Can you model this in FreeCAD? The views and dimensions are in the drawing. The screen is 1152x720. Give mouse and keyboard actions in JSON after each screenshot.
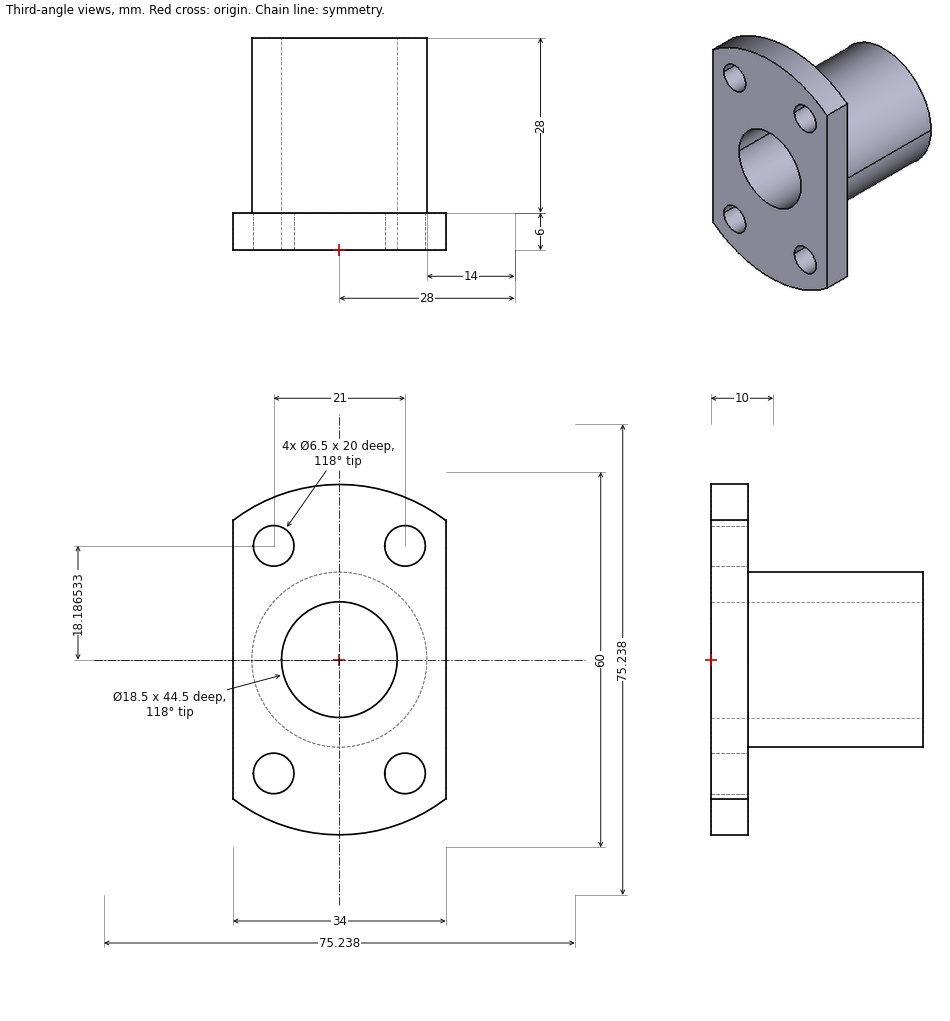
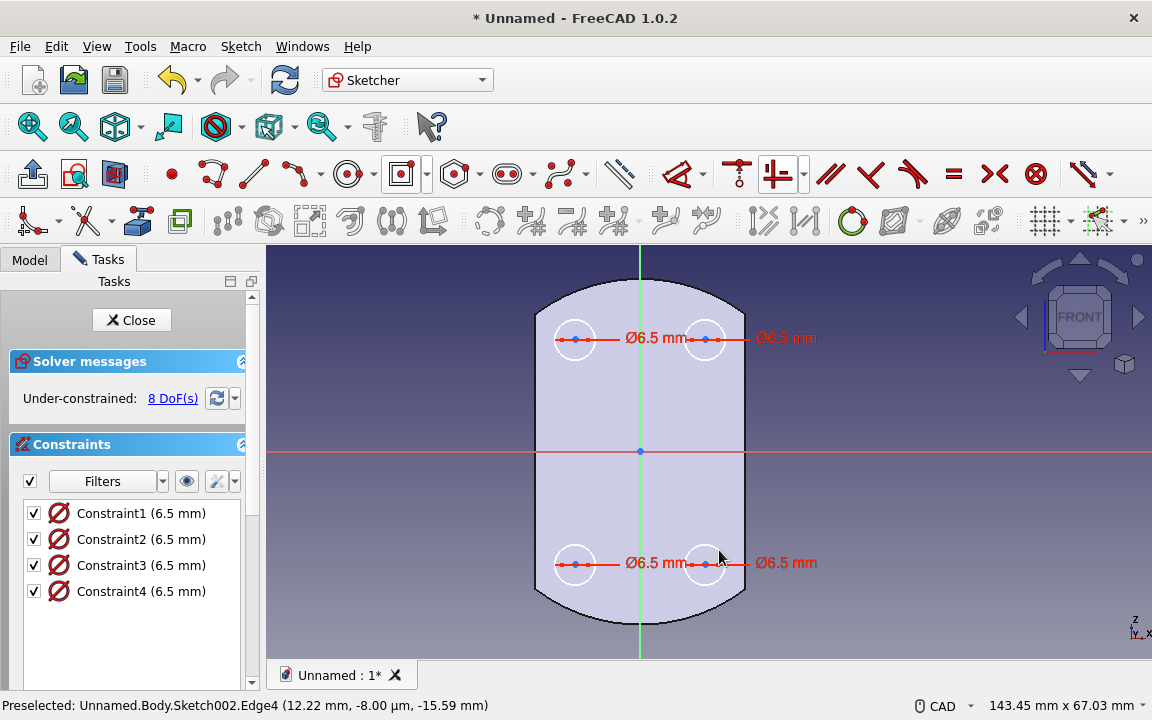
{"action": "left_click", "coordinate": [575, 340]}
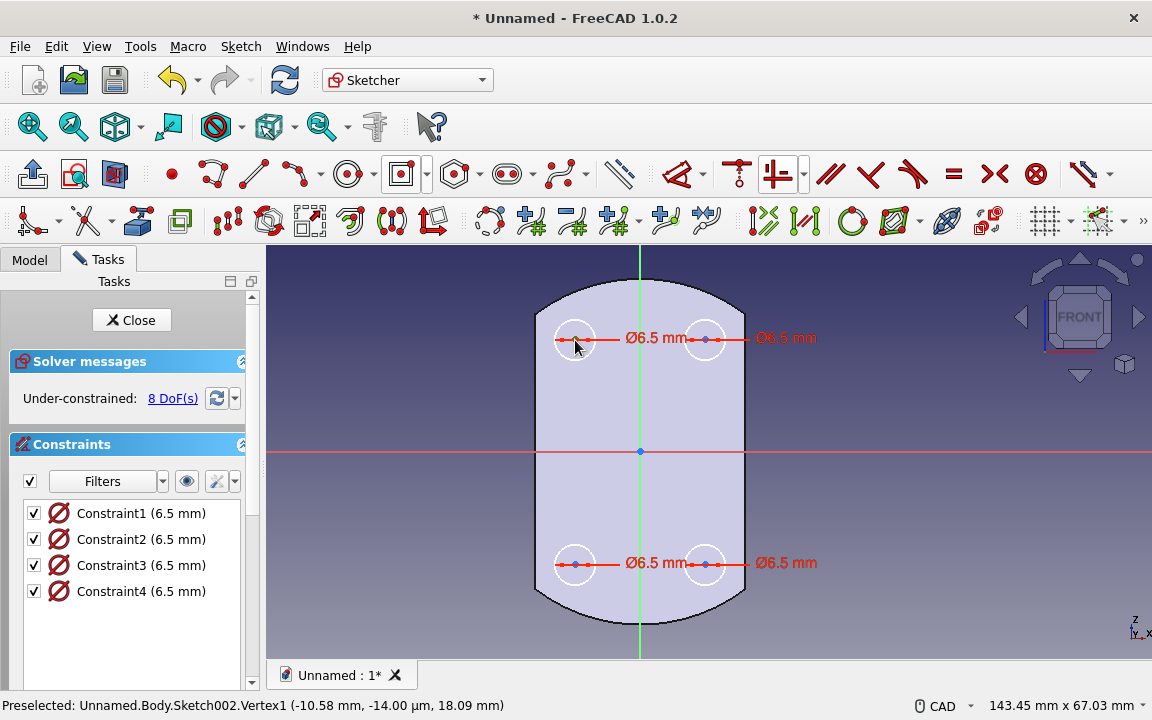
{"action": "left_click", "coordinate": [705, 340]}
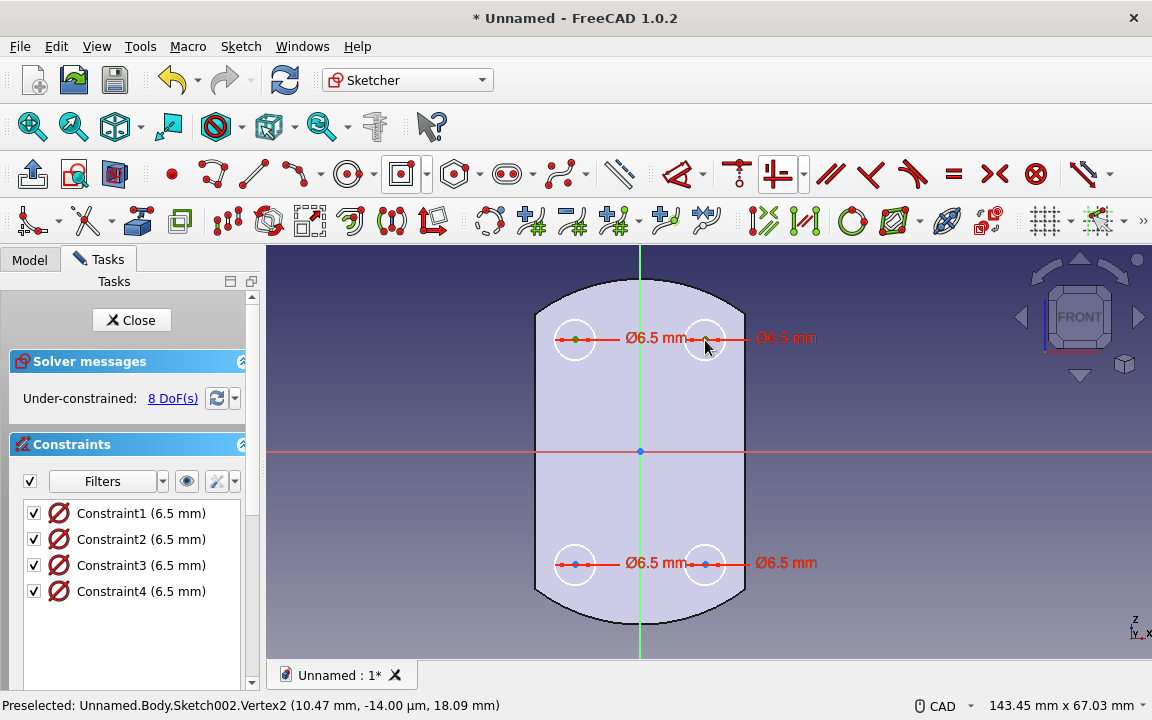
{"action": "left_click", "coordinate": [640, 605]}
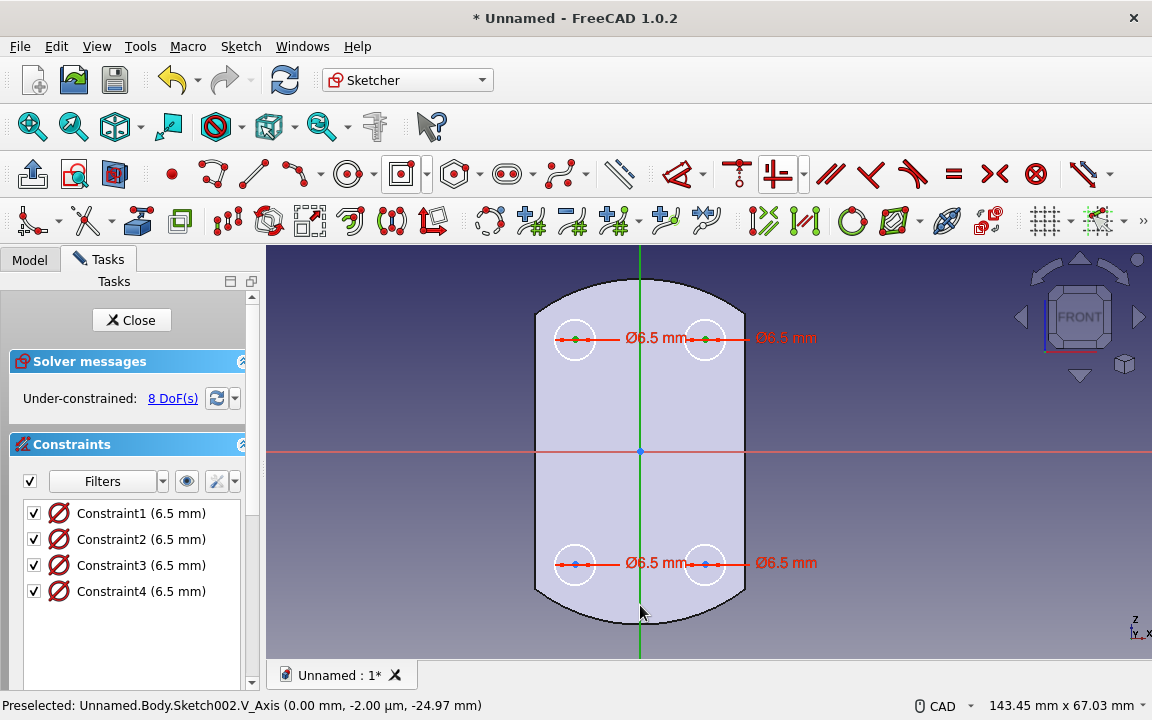
{"action": "left_click", "coordinate": [995, 174]}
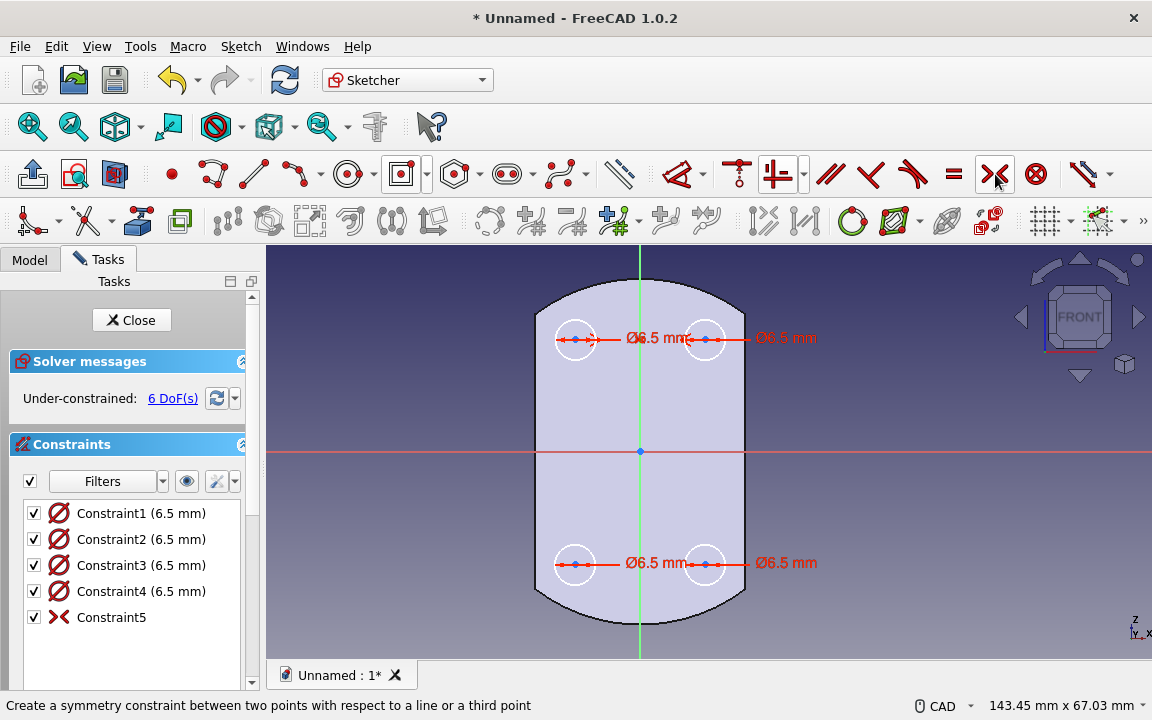
{"action": "left_click", "coordinate": [576, 340]}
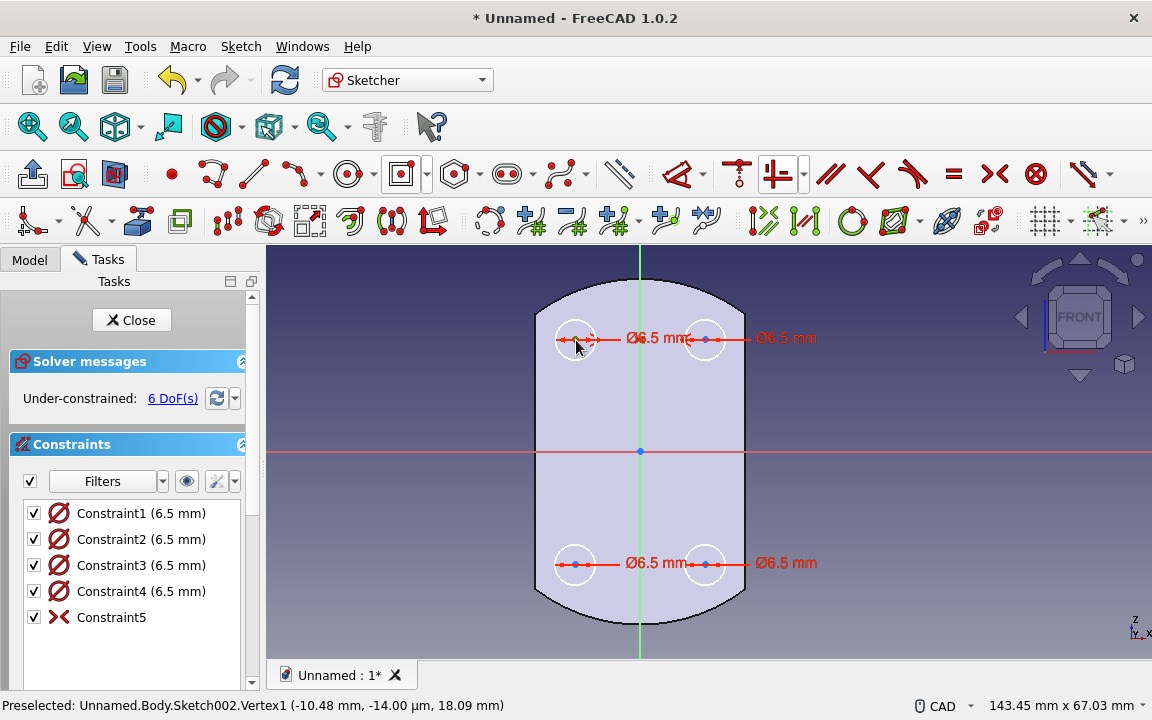
{"action": "left_click", "coordinate": [575, 565]}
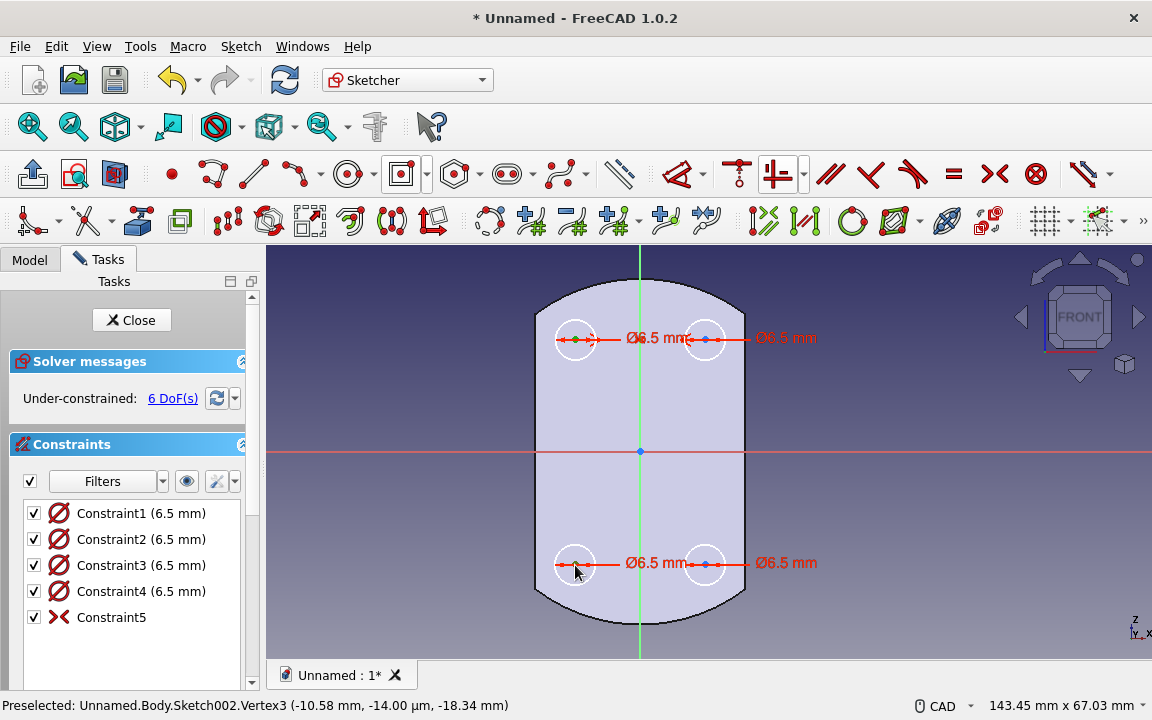
{"action": "left_click", "coordinate": [344, 452]}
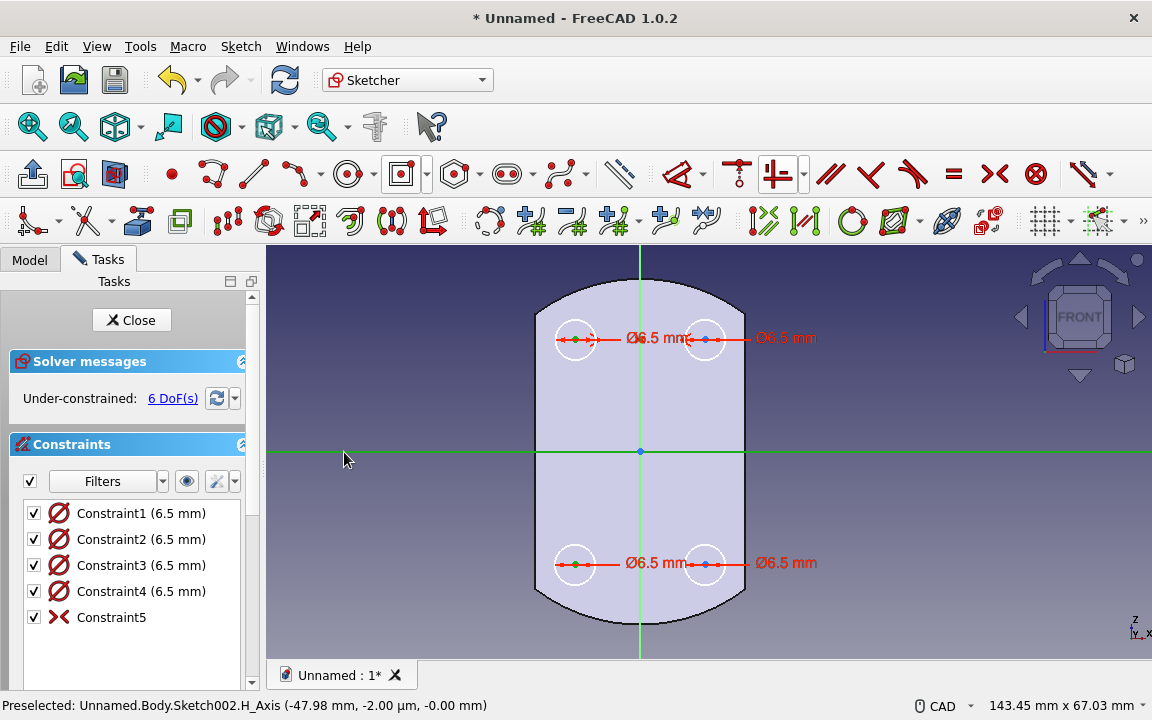
{"action": "left_click", "coordinate": [995, 174]}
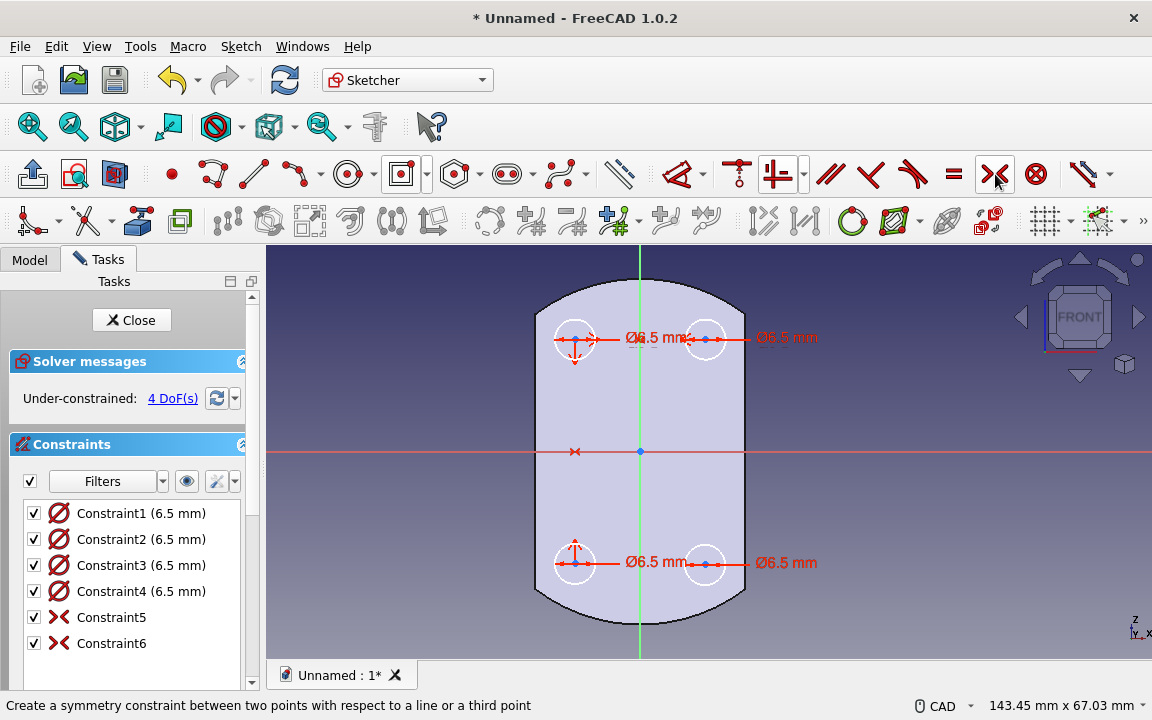
{"action": "left_click", "coordinate": [706, 340]}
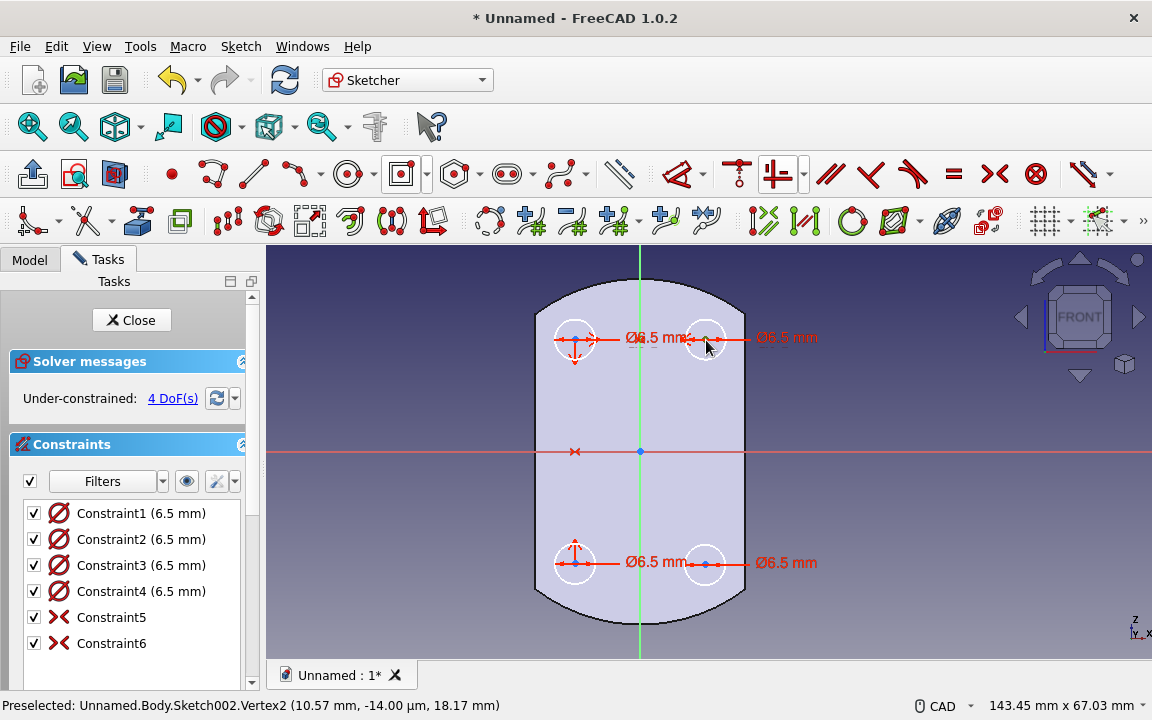
{"action": "left_click", "coordinate": [705, 565]}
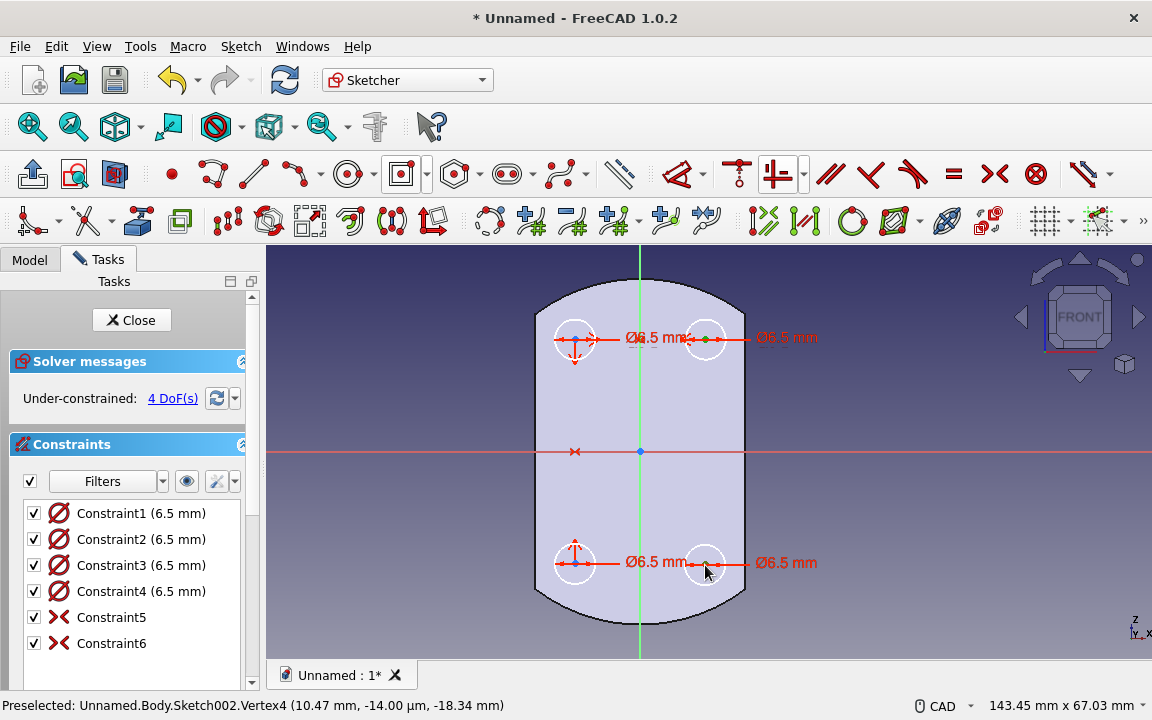
{"action": "left_click", "coordinate": [344, 452]}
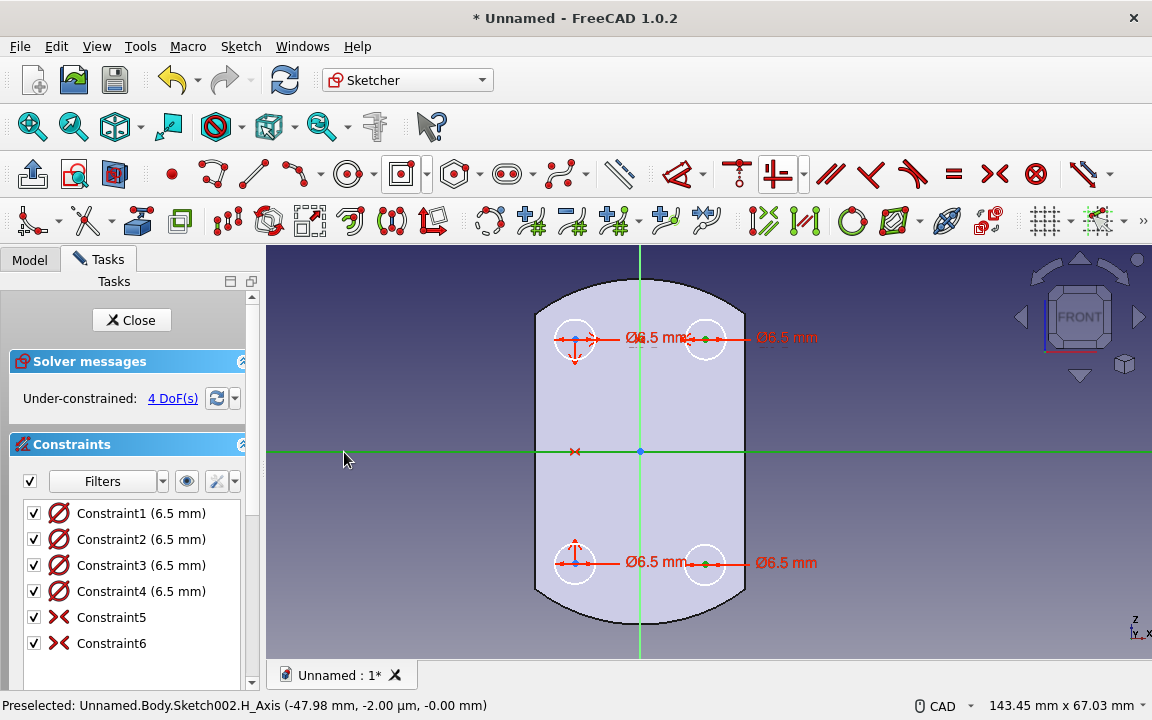
{"action": "left_click", "coordinate": [995, 174]}